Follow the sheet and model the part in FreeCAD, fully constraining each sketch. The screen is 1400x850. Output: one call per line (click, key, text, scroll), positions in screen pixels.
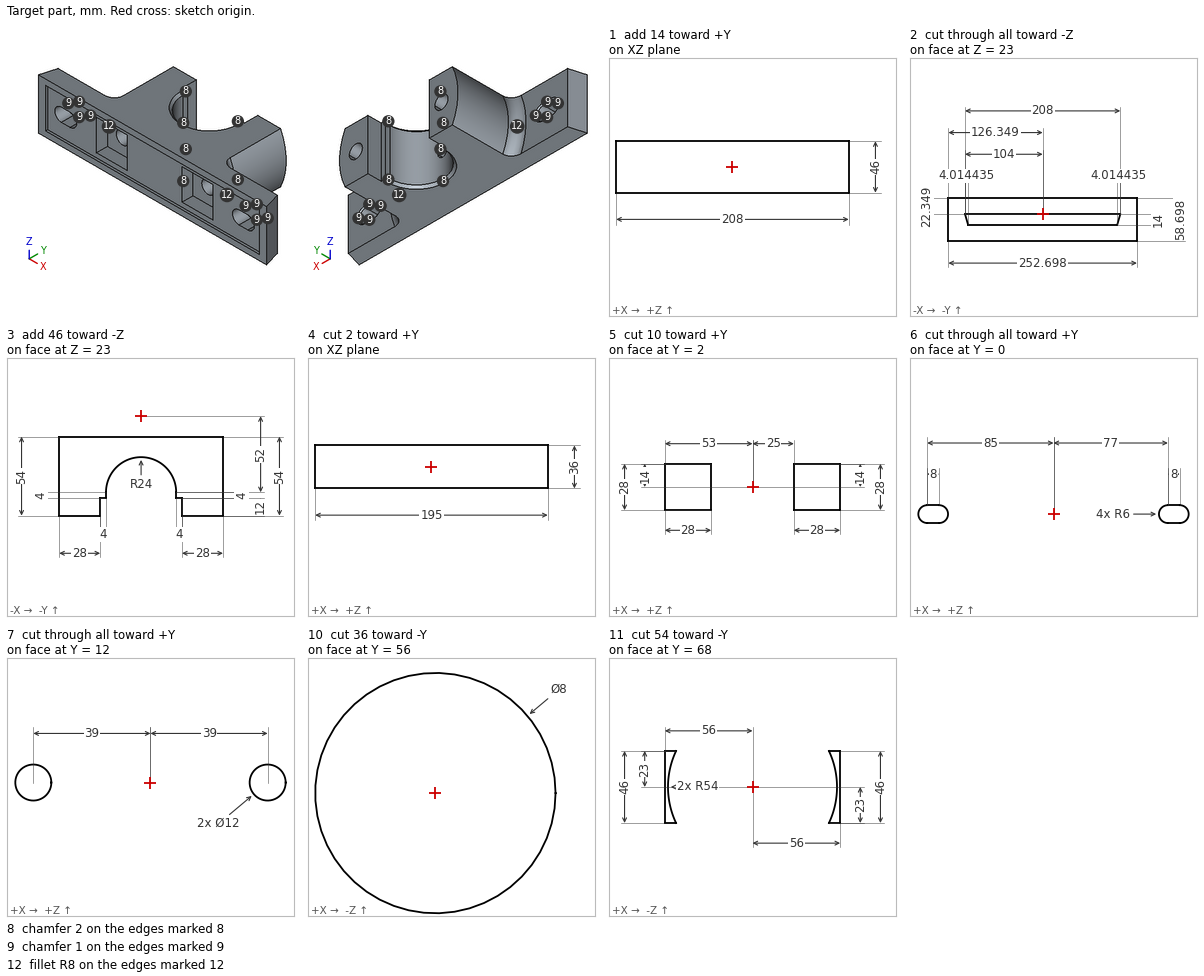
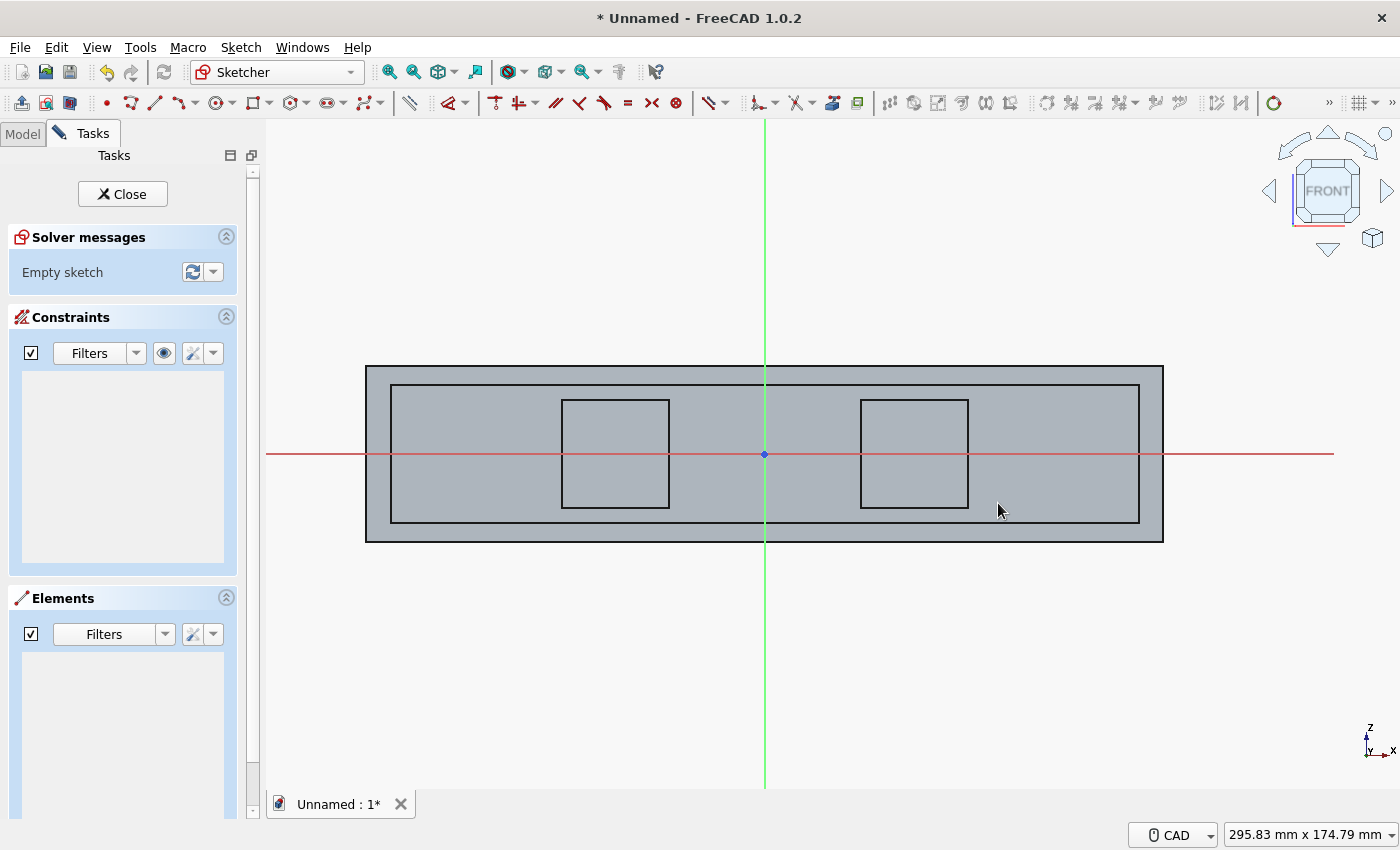
click(1060, 454)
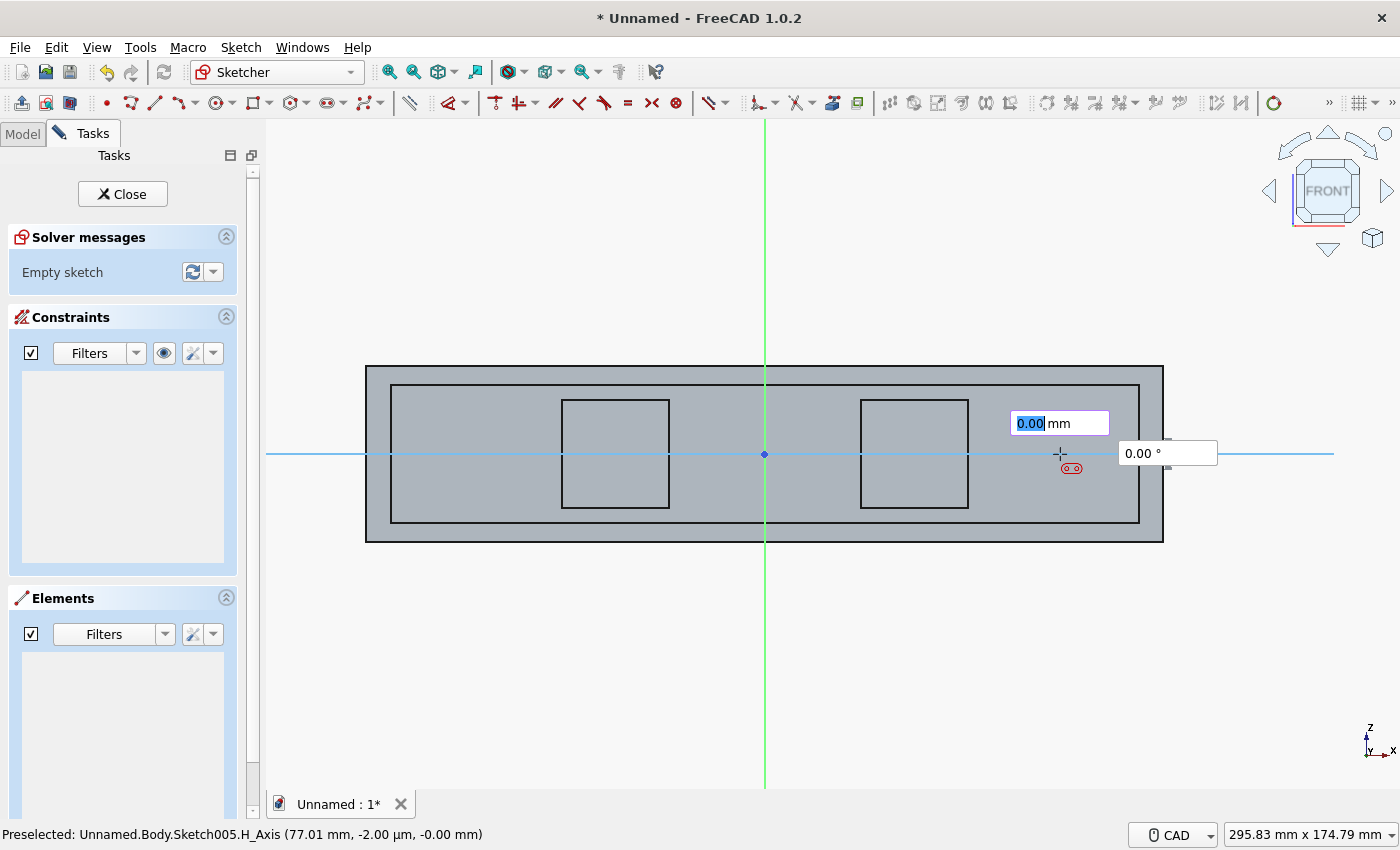
click(1091, 445)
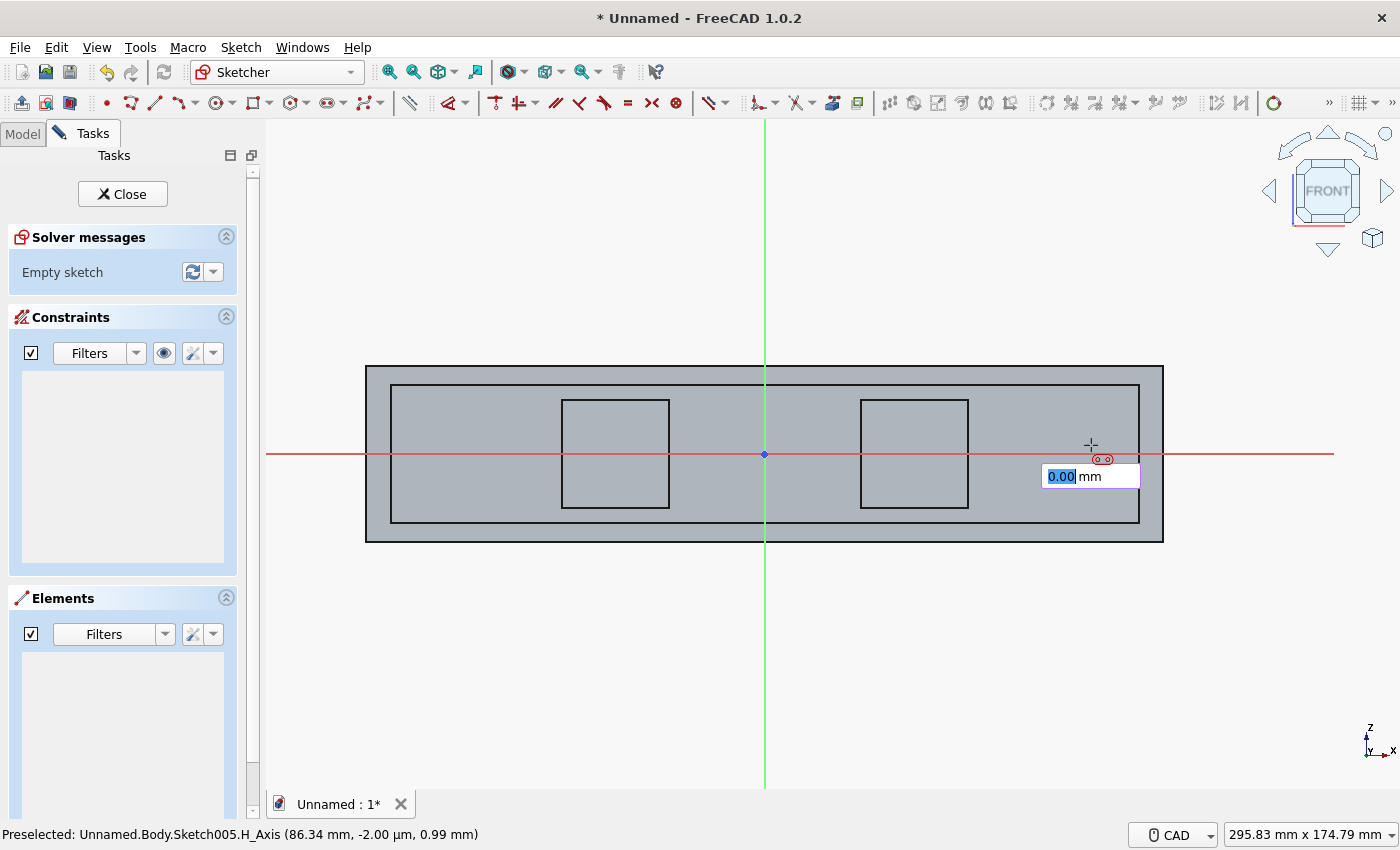
click(1075, 477)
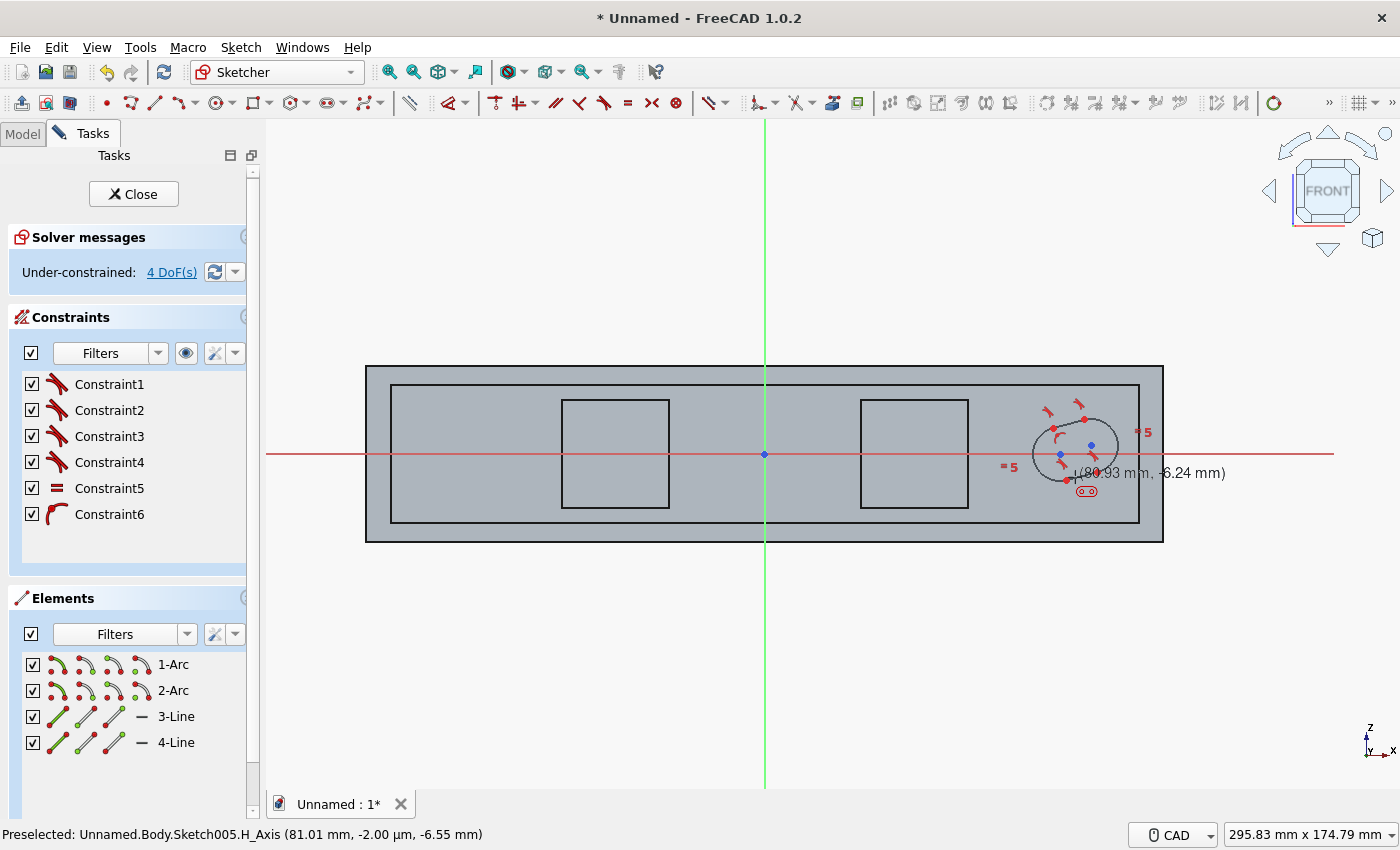
click(439, 454)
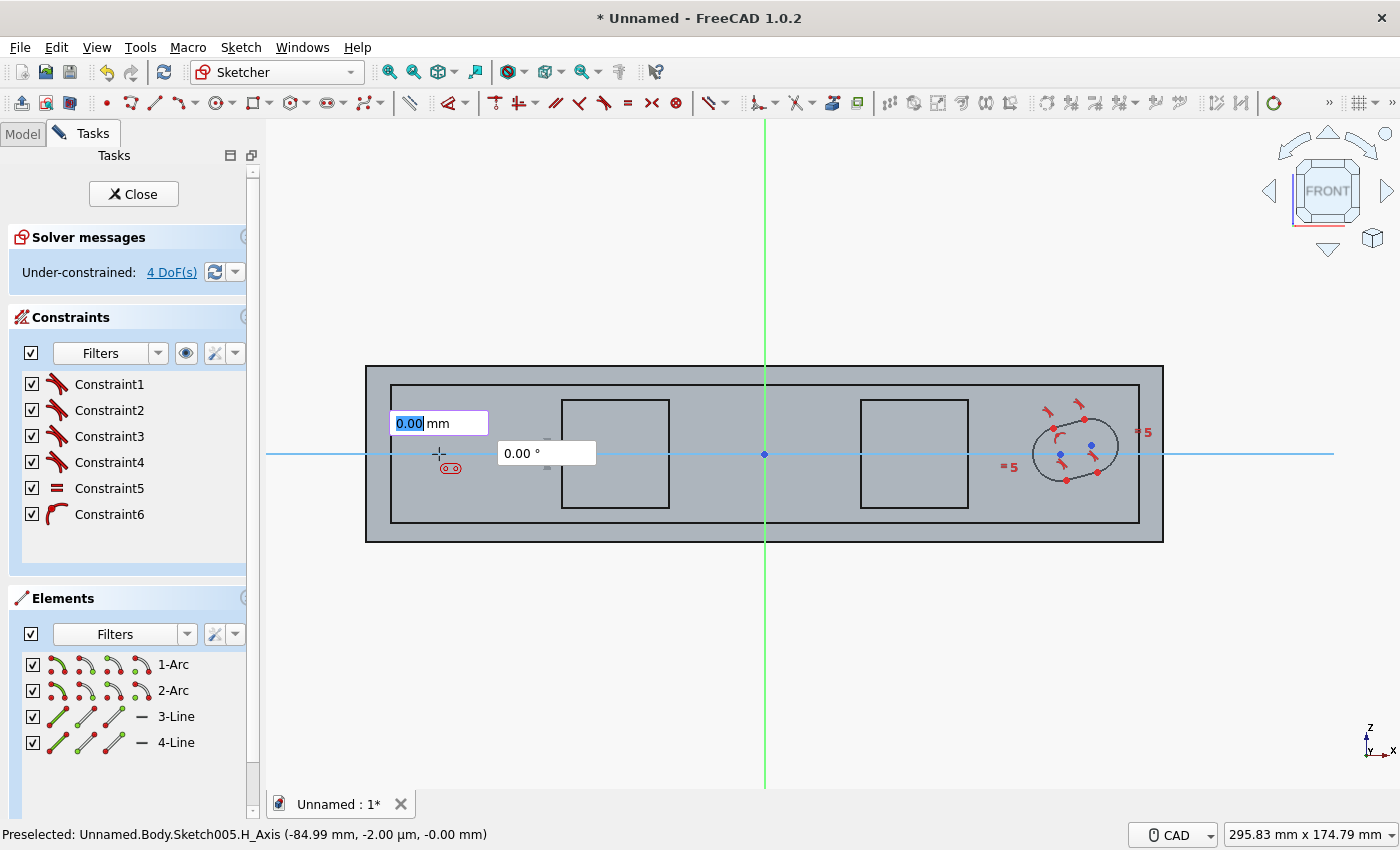
click(470, 445)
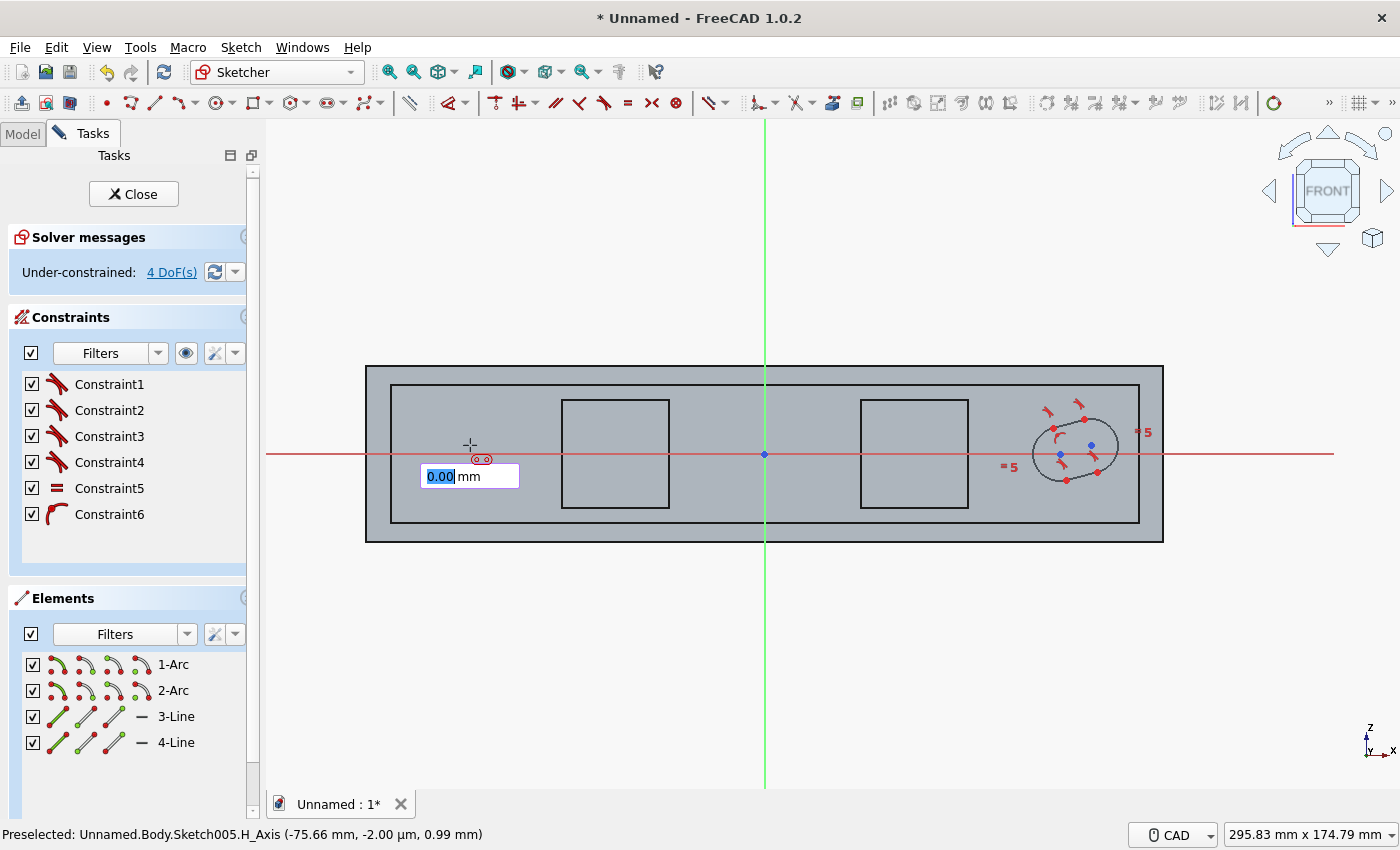
click(454, 477)
key(Escape)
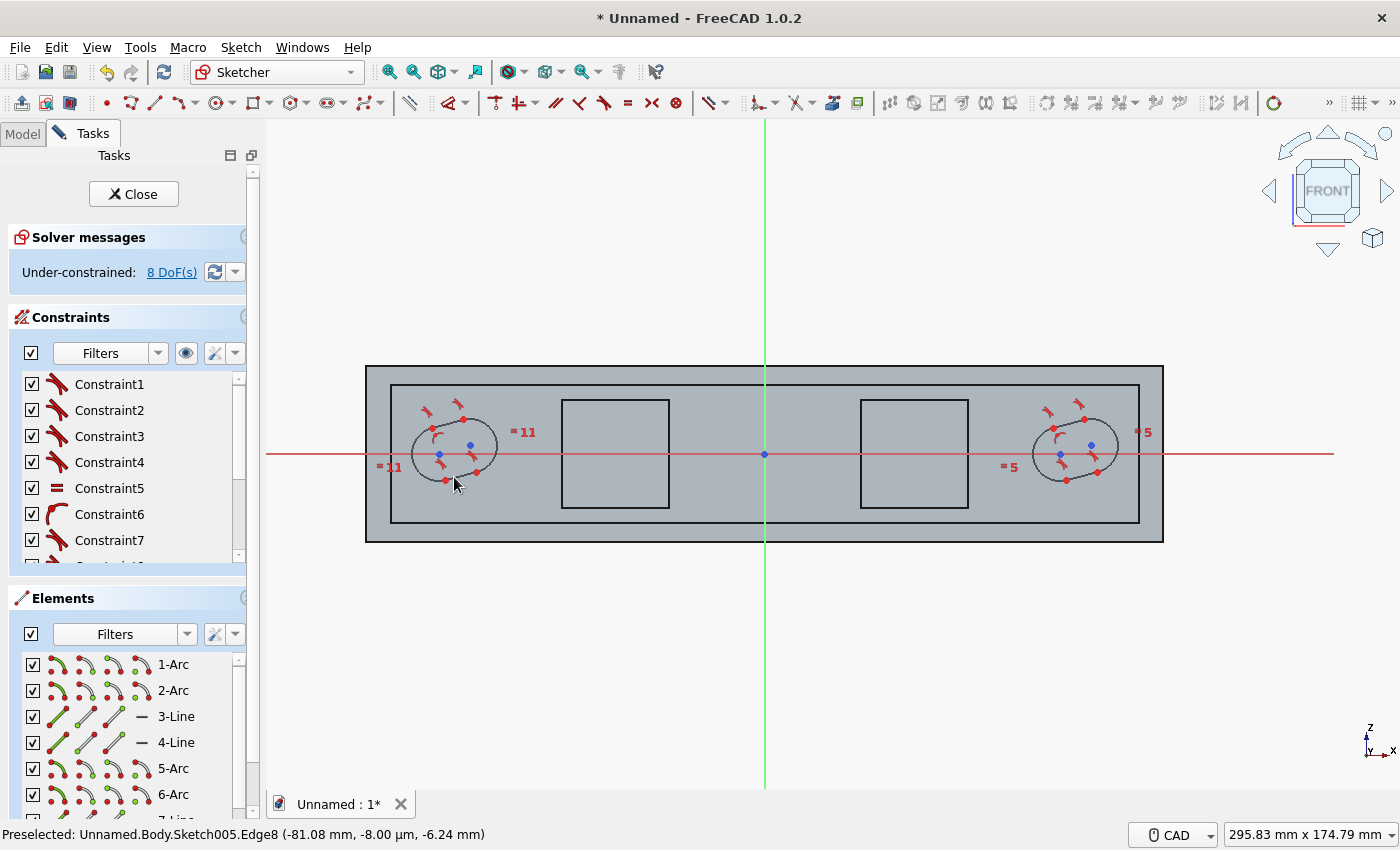
scroll(1063, 426, up, 2)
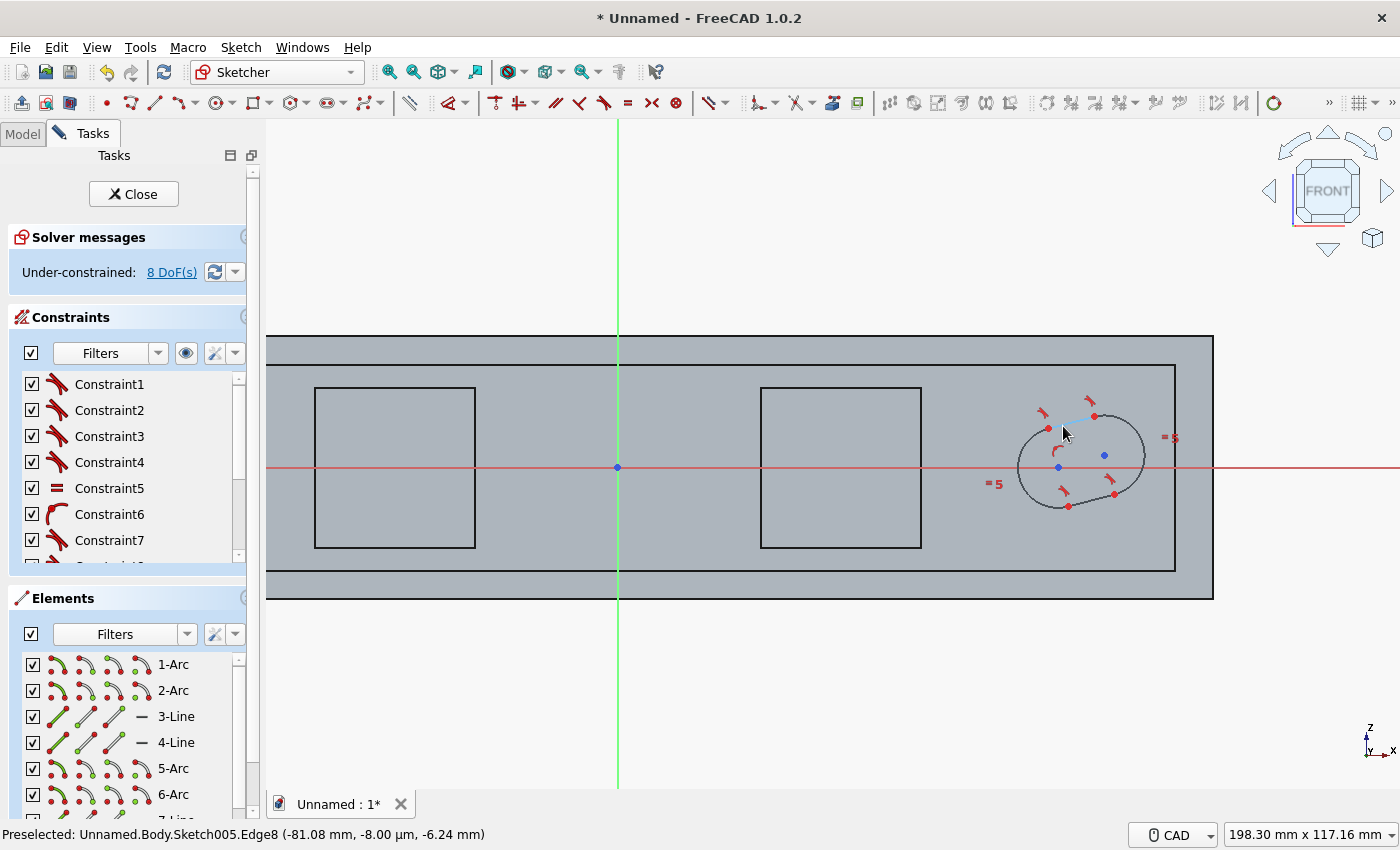
click(1062, 425)